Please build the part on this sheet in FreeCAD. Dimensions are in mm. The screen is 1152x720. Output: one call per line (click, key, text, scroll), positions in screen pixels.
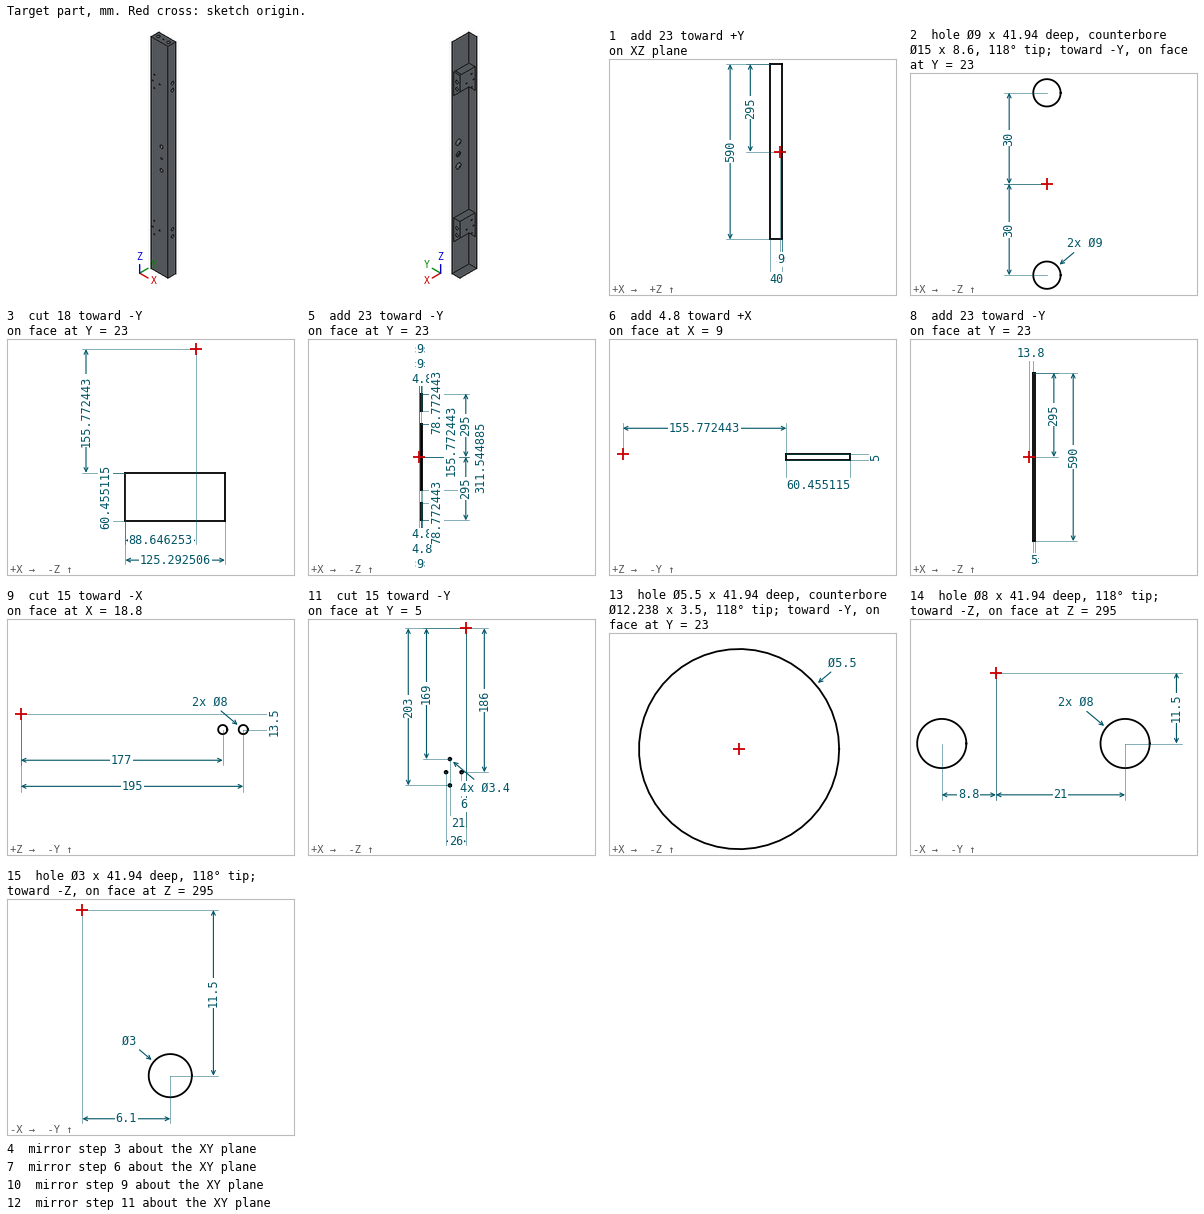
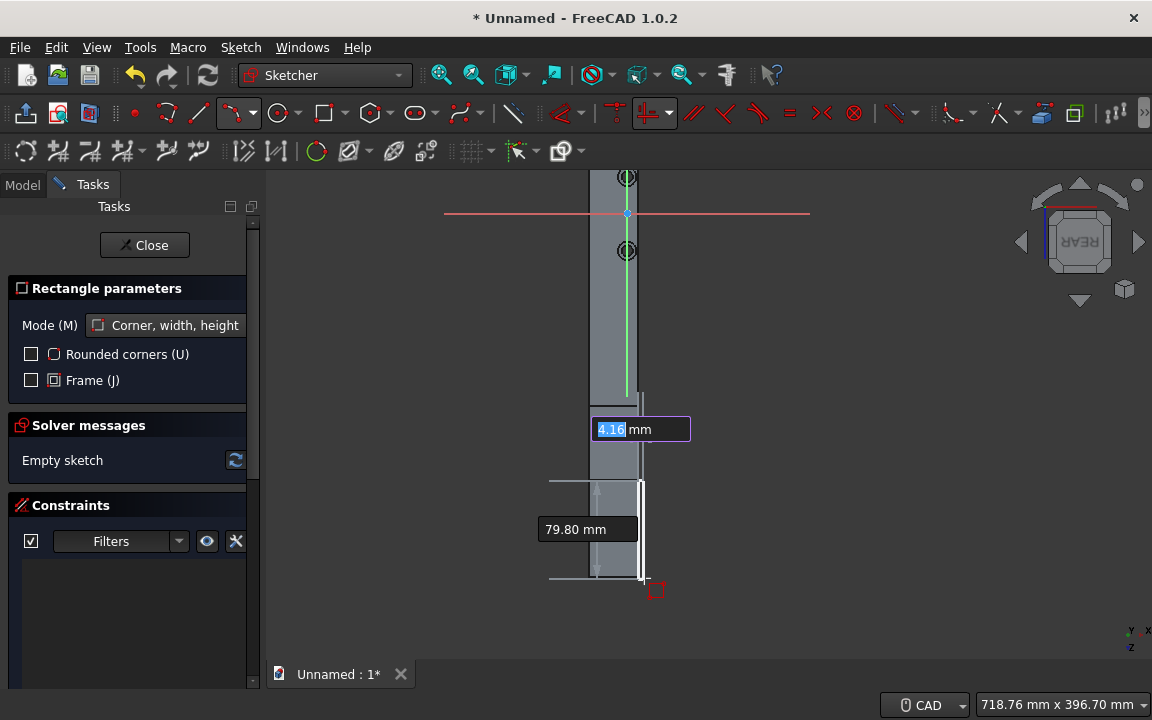
click(644, 577)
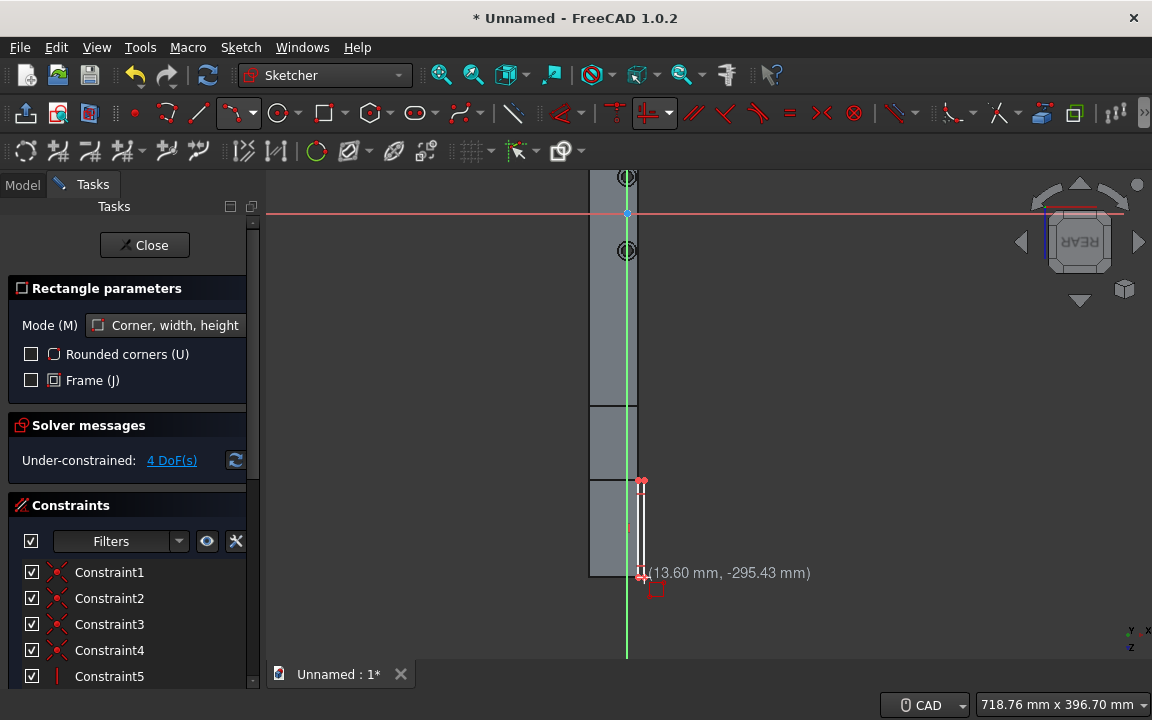
scroll(644, 578, down, 4)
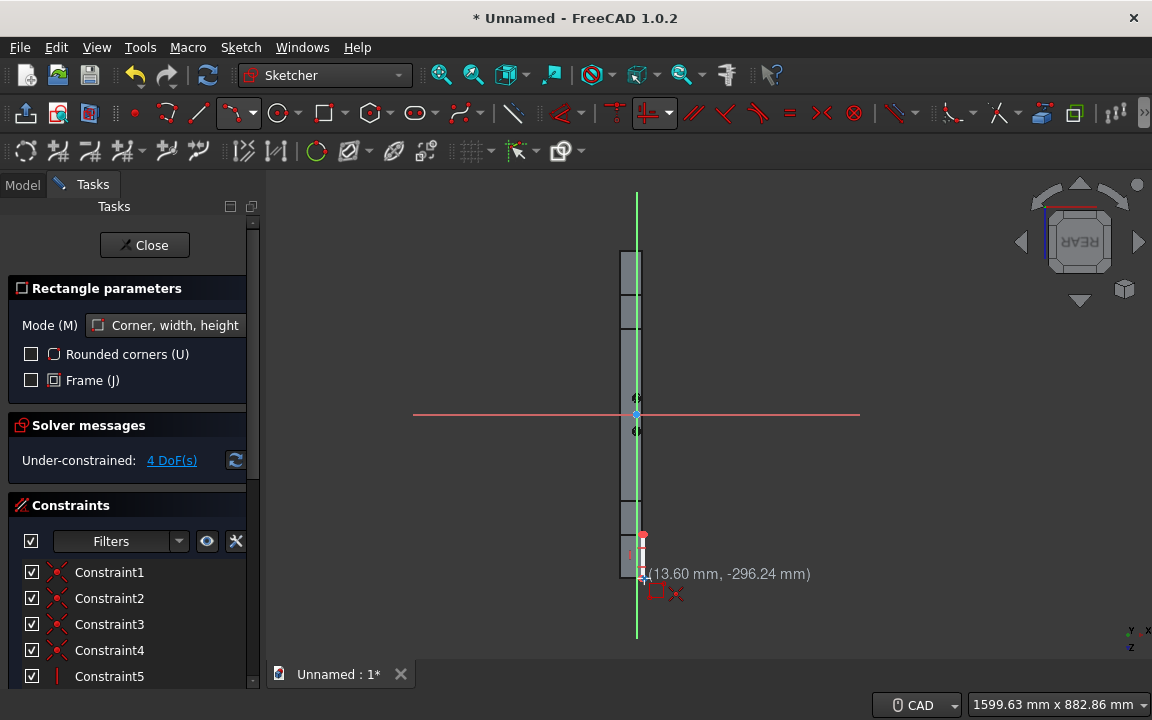
scroll(642, 251, up, 9)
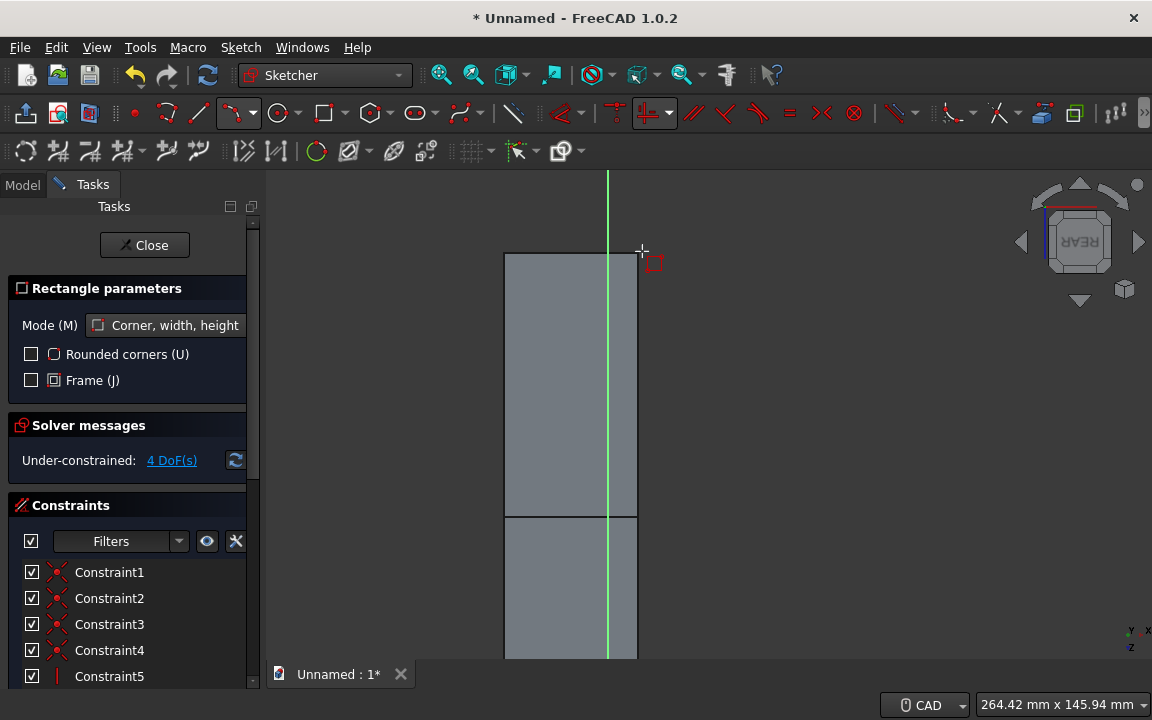
click(638, 253)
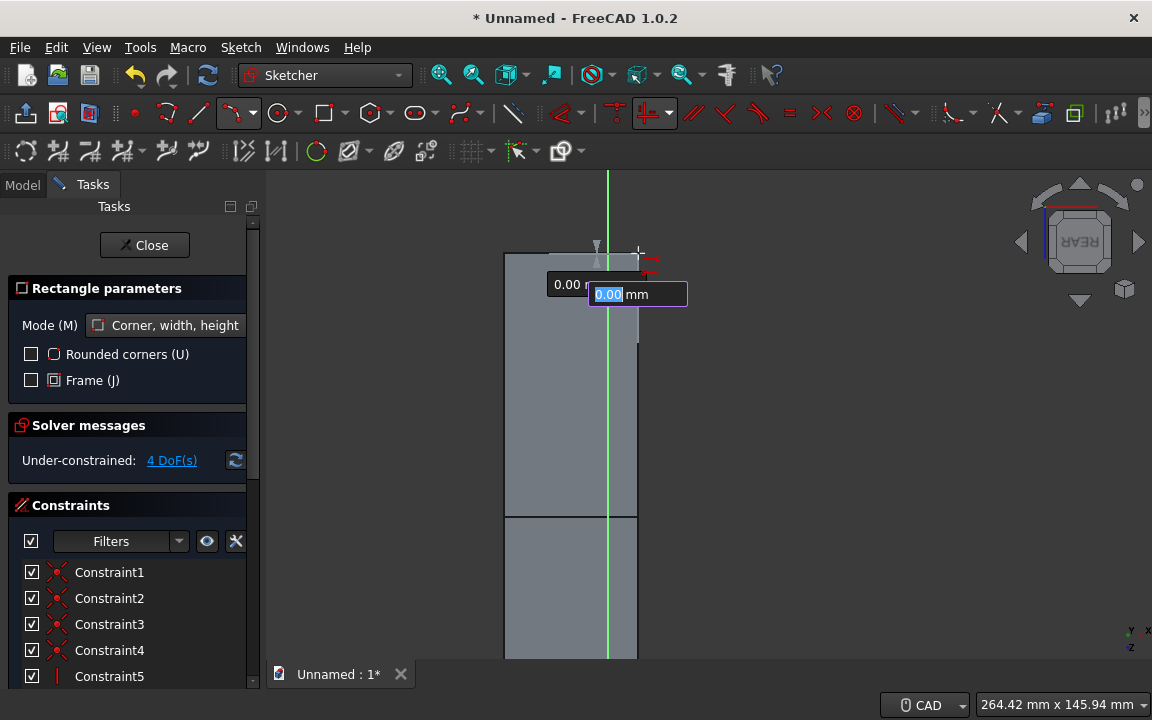
scroll(642, 251, down, 9)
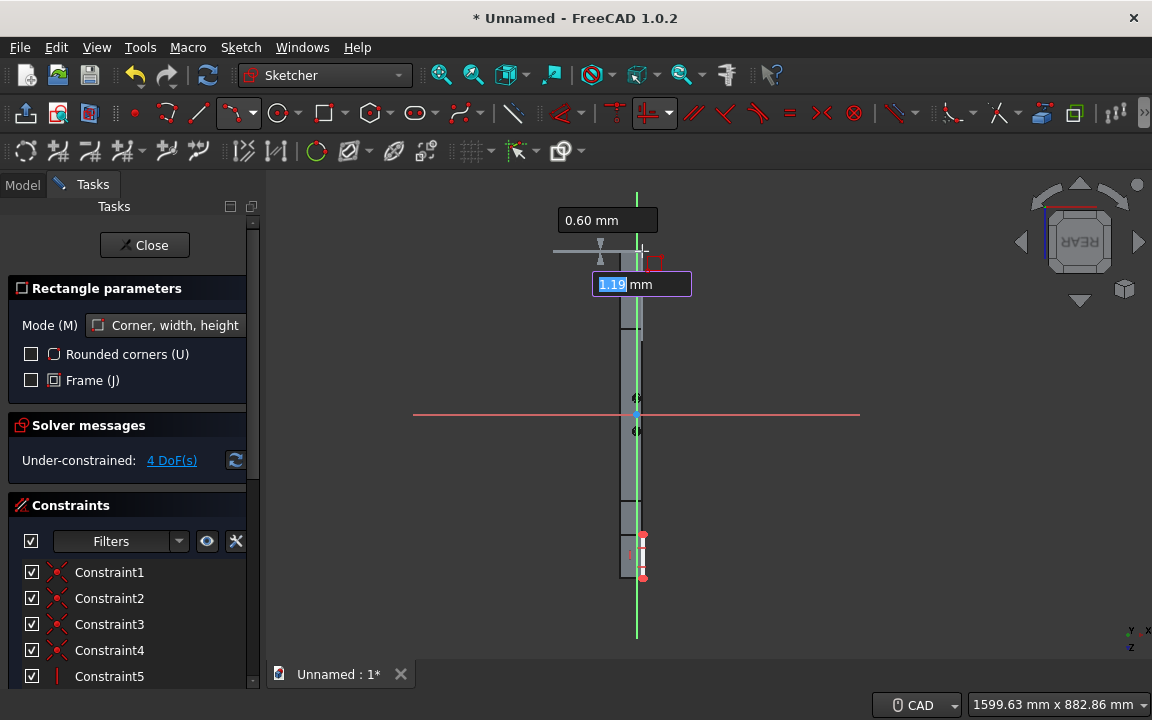
scroll(644, 295, up, 4)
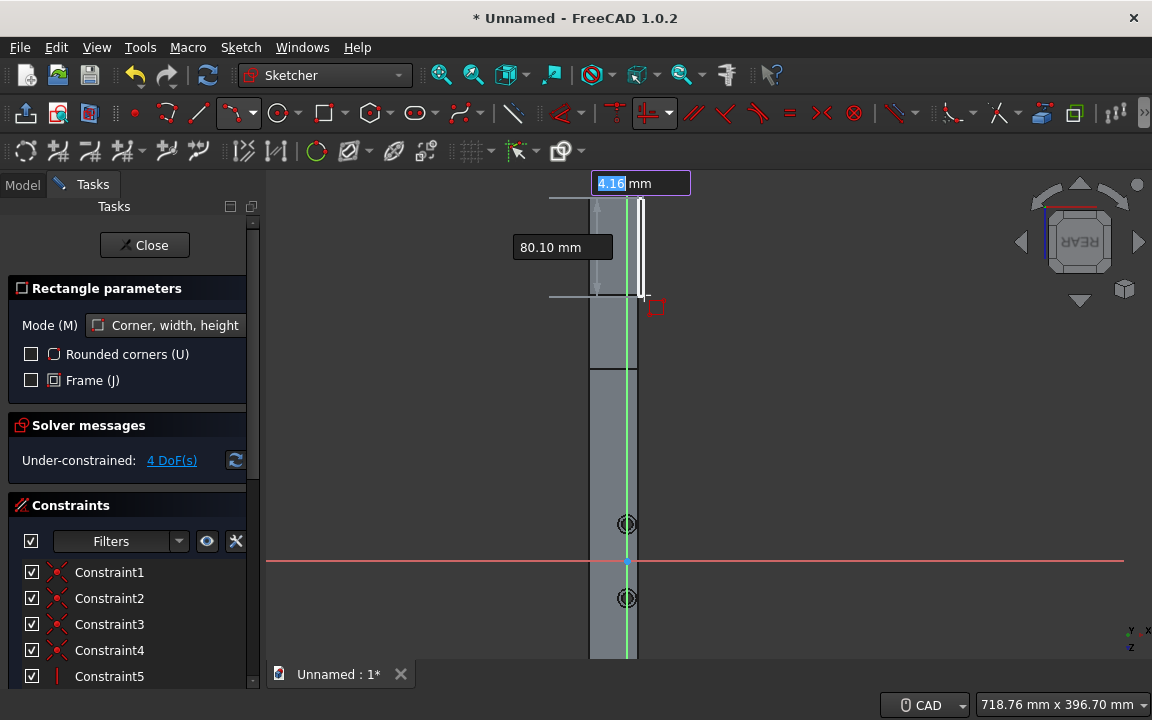
click(644, 295)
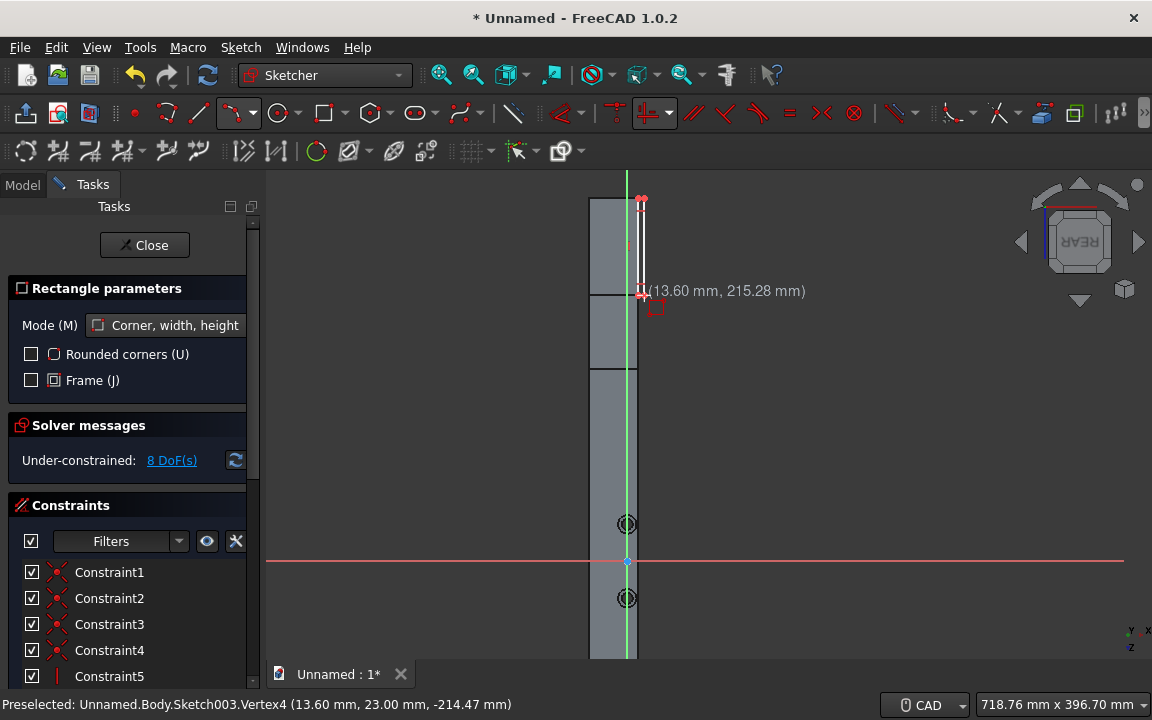
scroll(638, 369, up, 5)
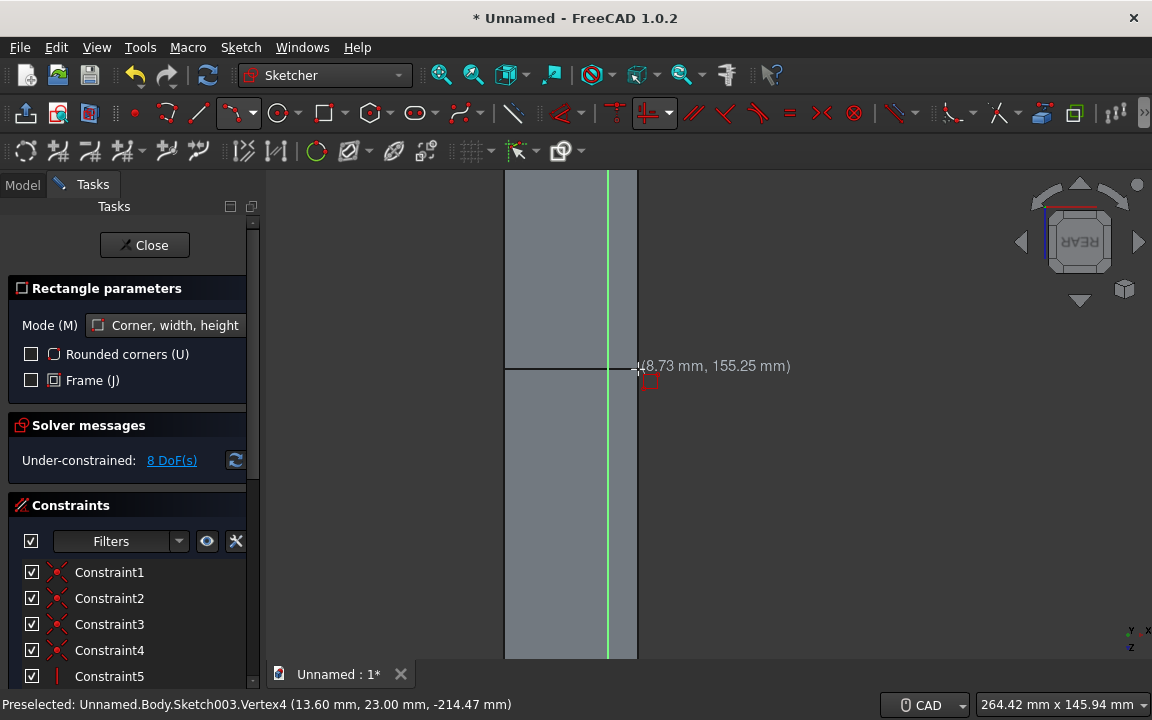
click(638, 369)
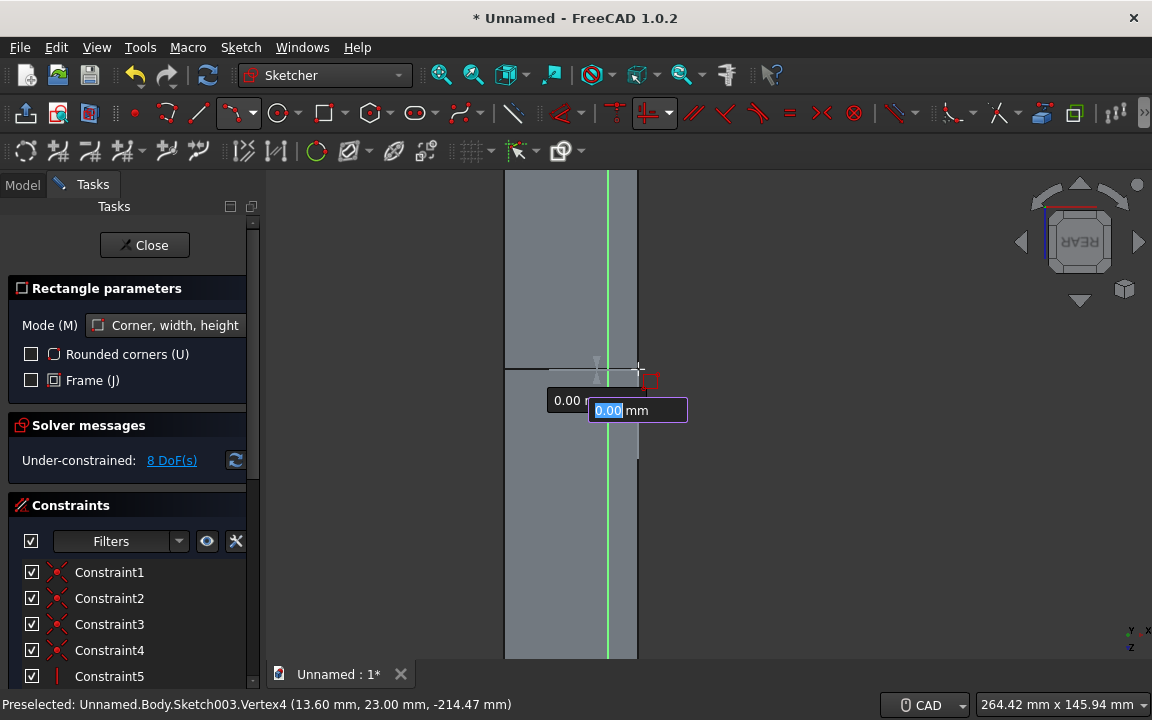
scroll(642, 320, down, 9)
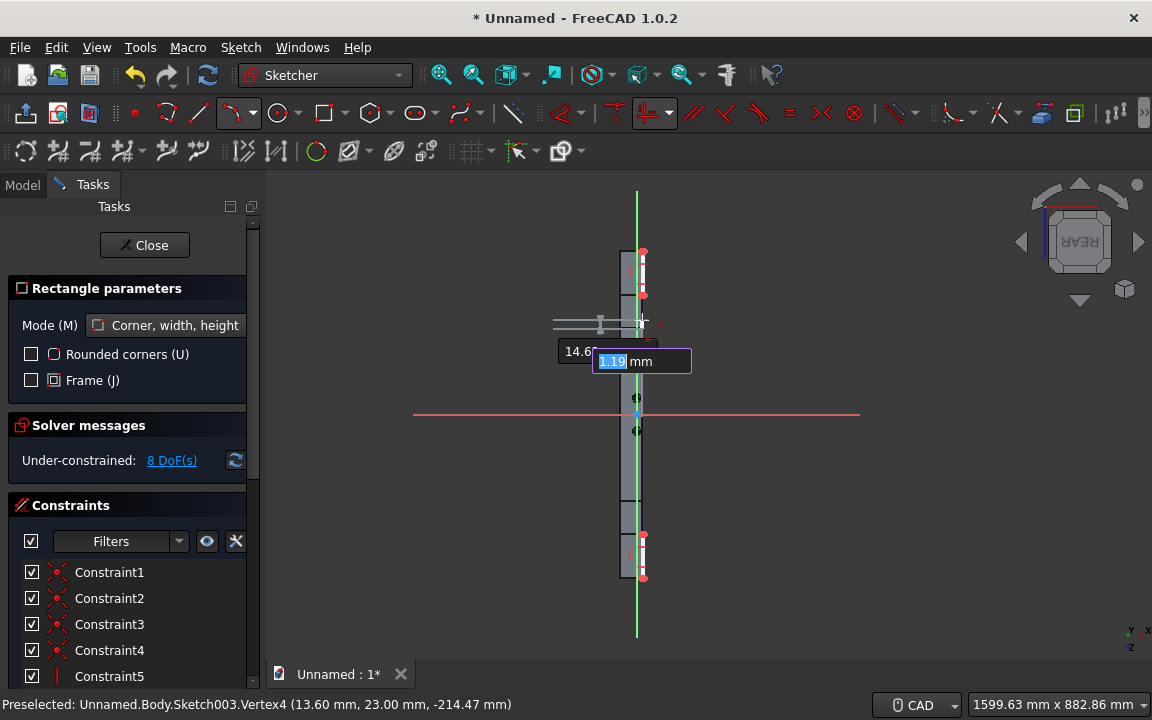
scroll(644, 501, up, 4)